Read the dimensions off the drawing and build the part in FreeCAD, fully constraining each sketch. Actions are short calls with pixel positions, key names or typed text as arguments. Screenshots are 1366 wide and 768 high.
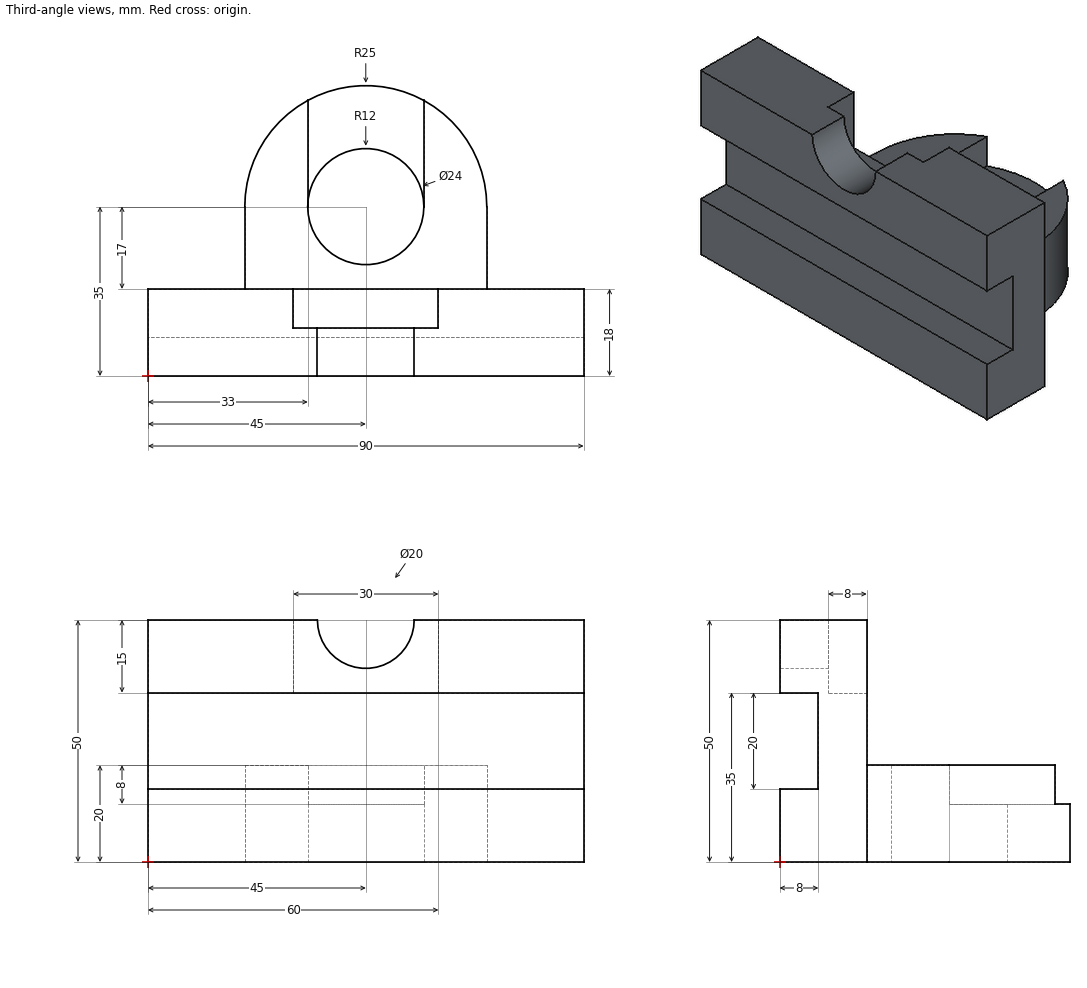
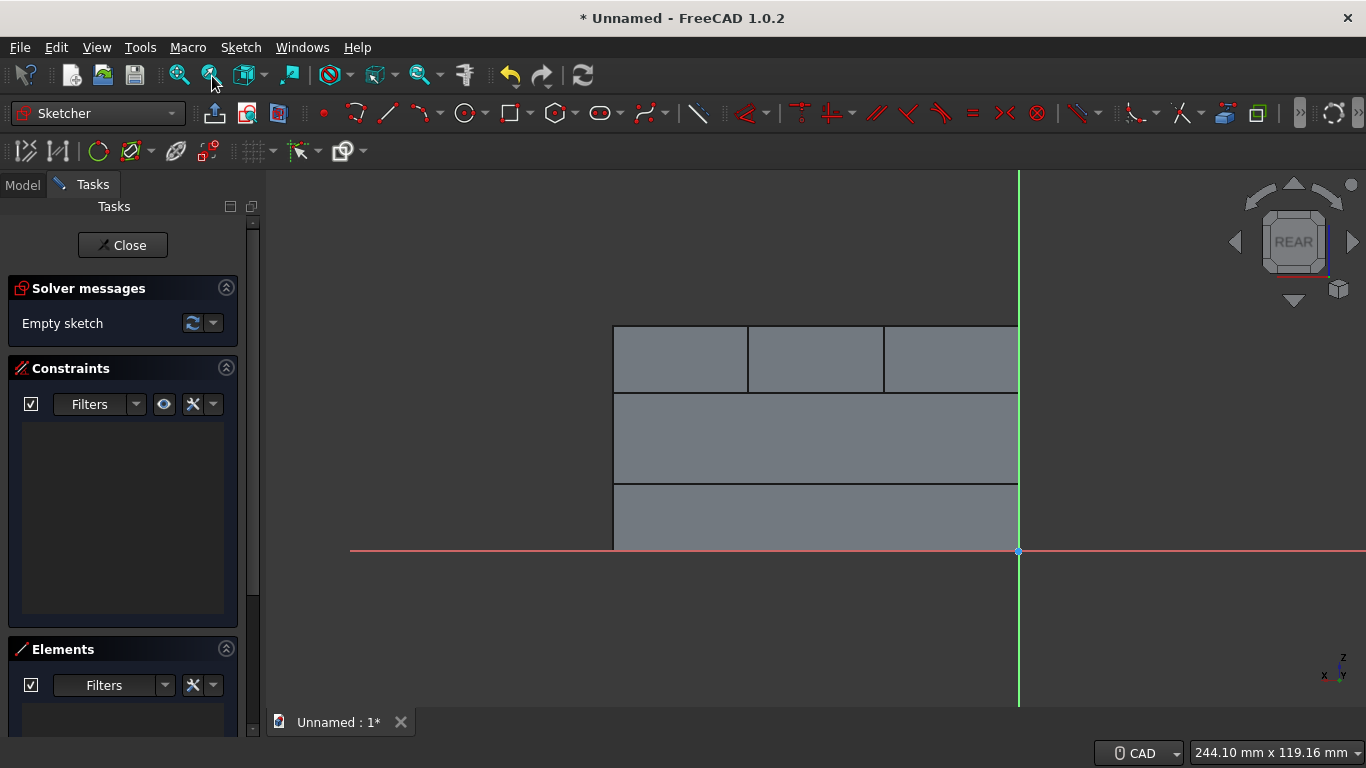
scroll(838, 289, up, 7)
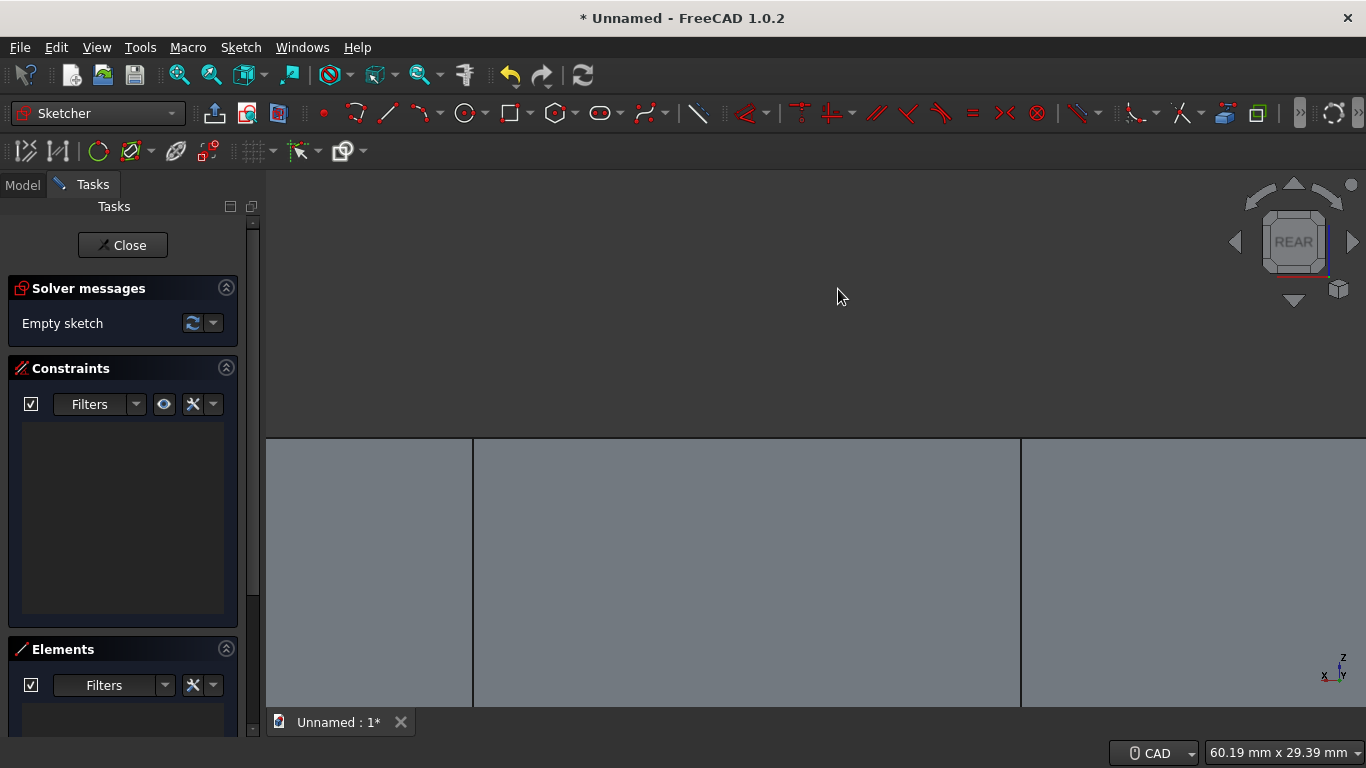
click(466, 114)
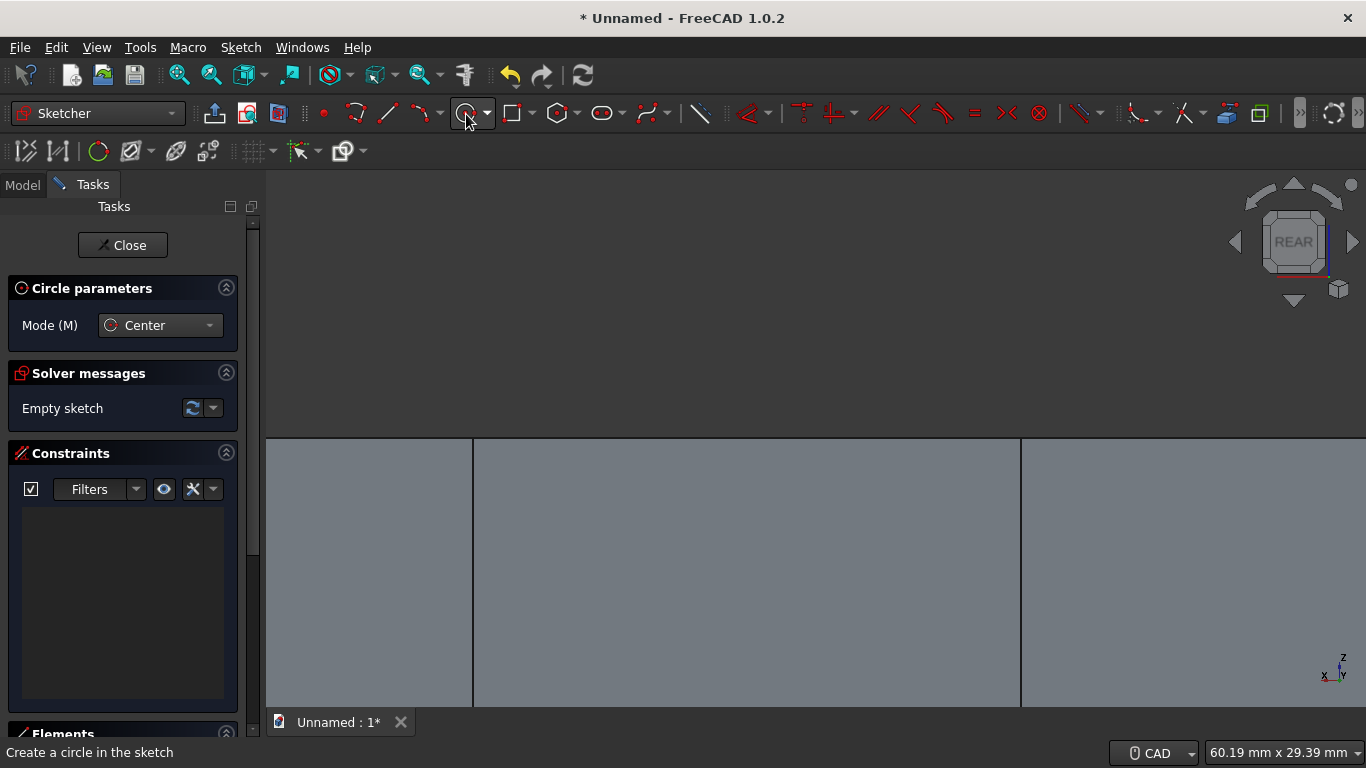
click(747, 438)
move(876, 308)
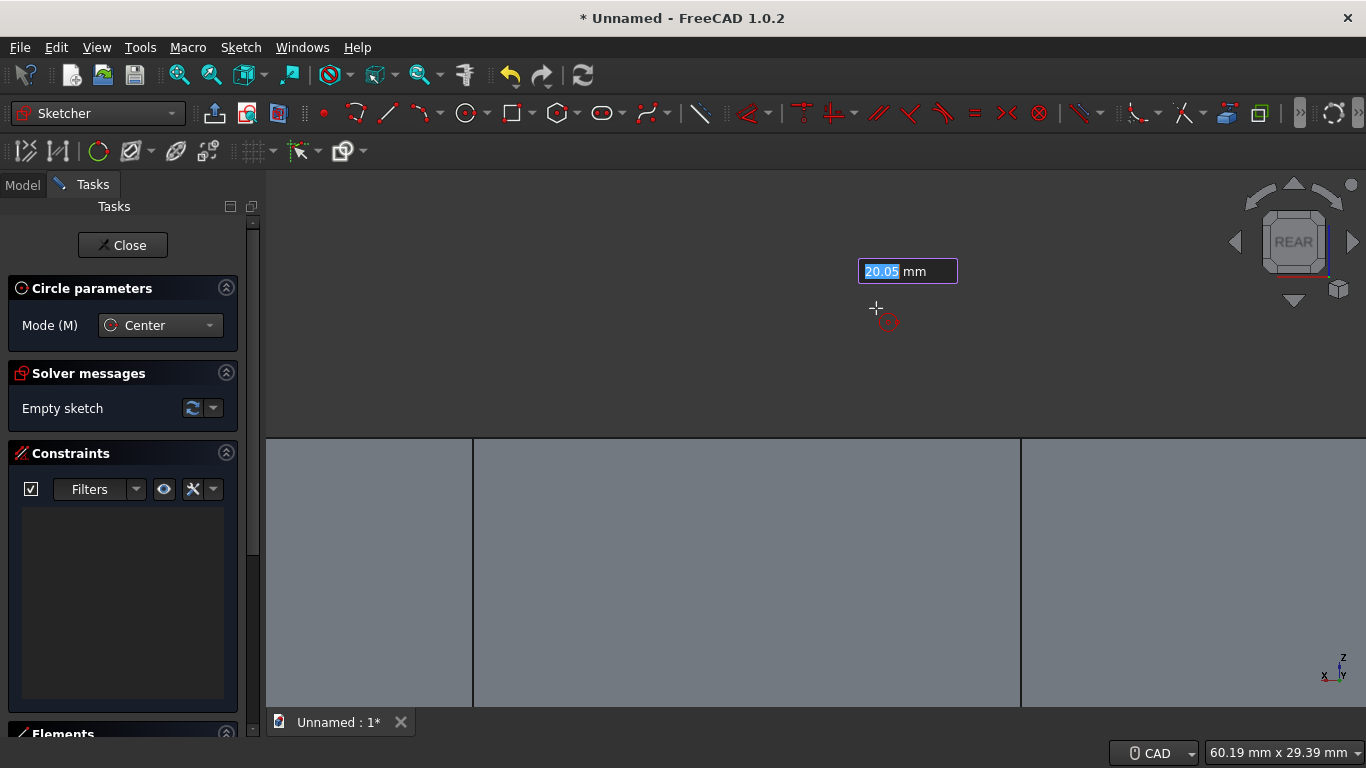
text(20)
key(Return)
key(Escape)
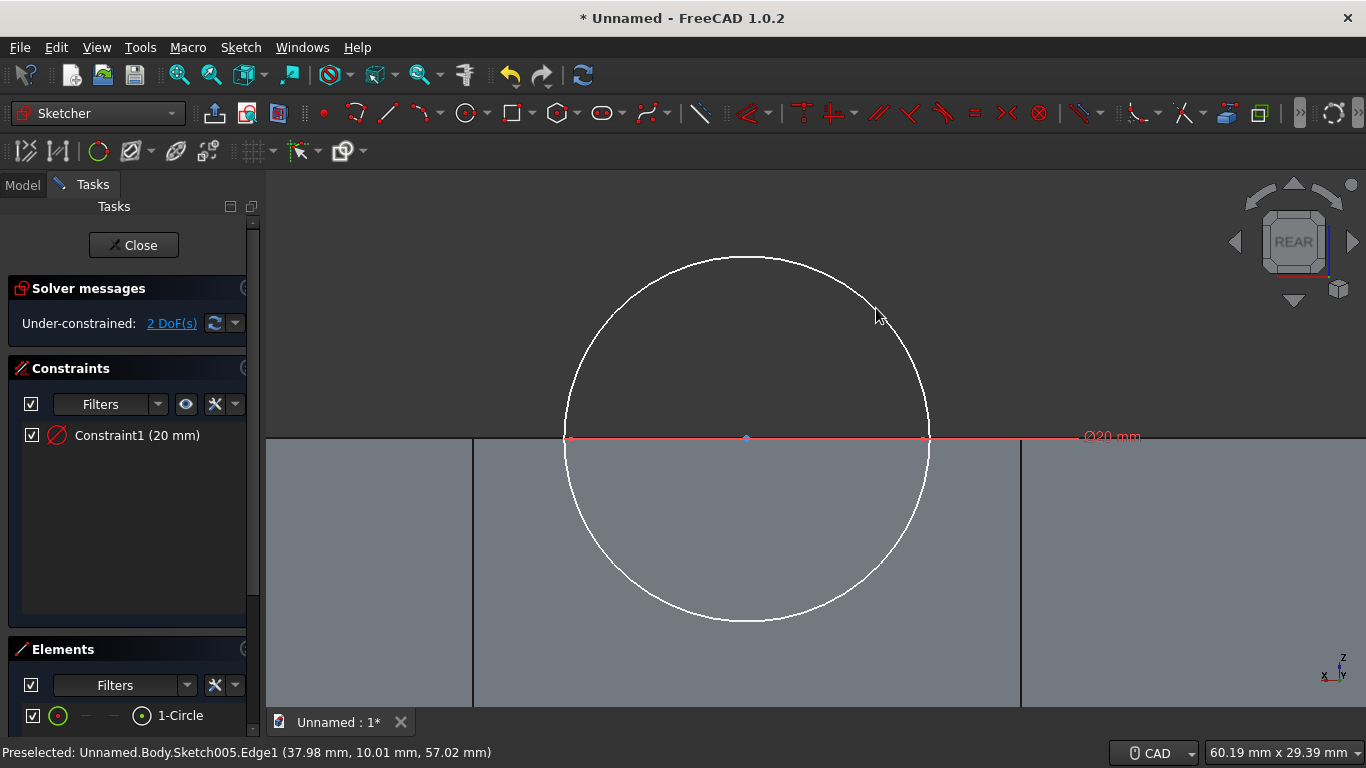
key(d)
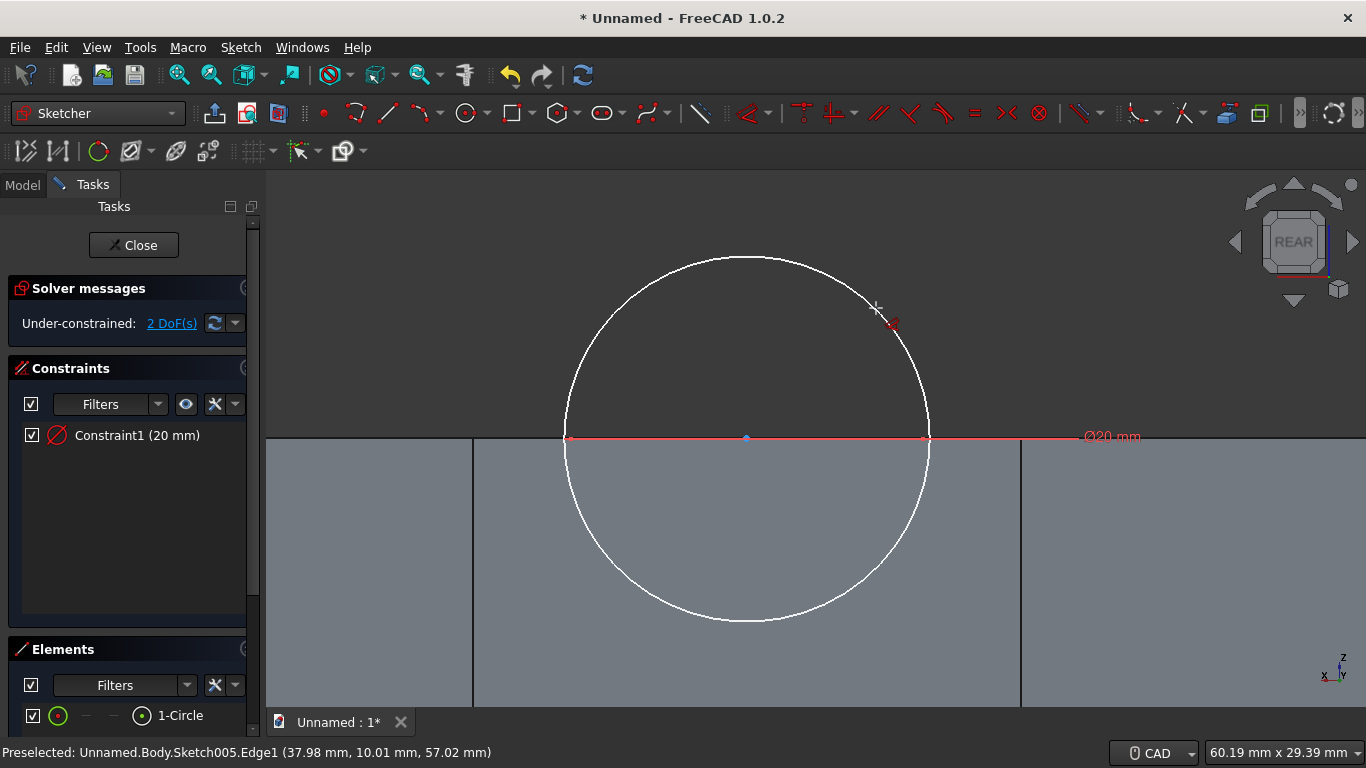
click(747, 439)
click(974, 405)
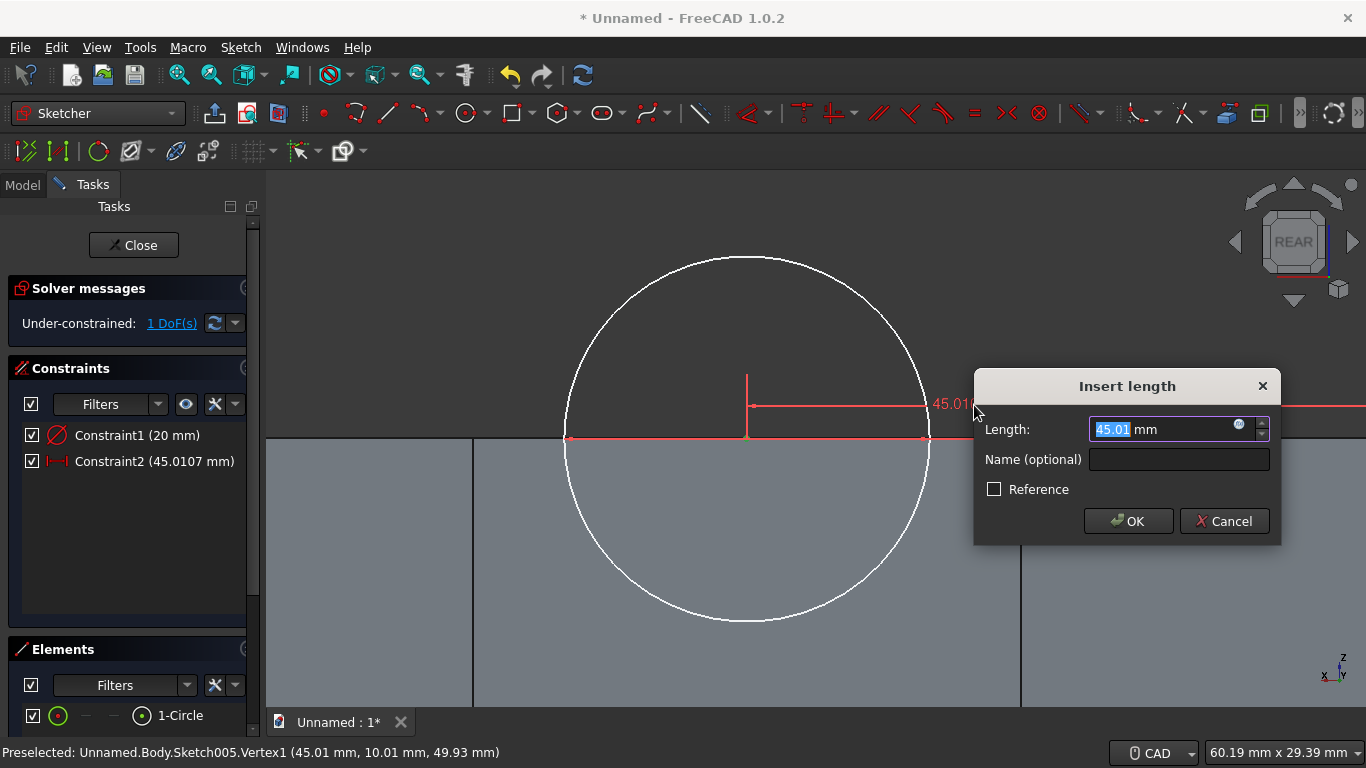
text(45)
key(Return)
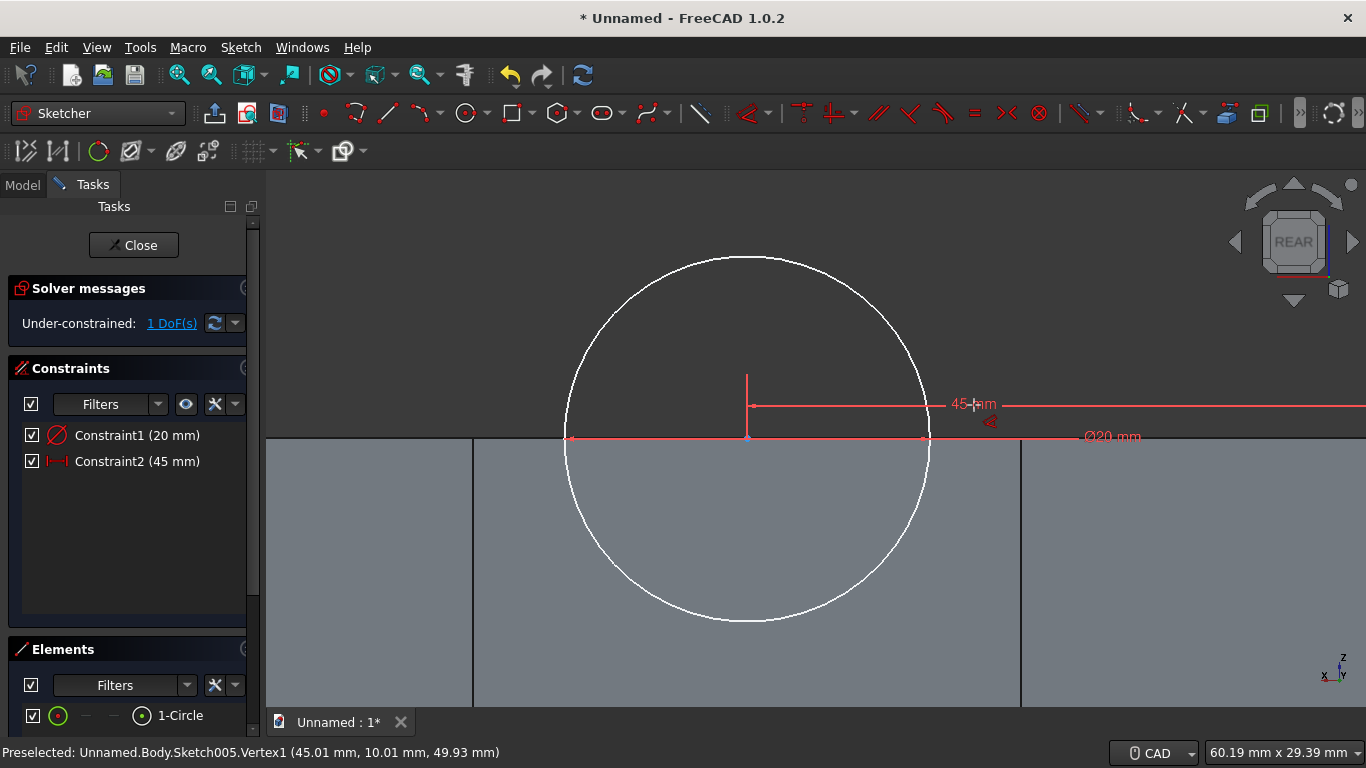
click(747, 439)
click(713, 559)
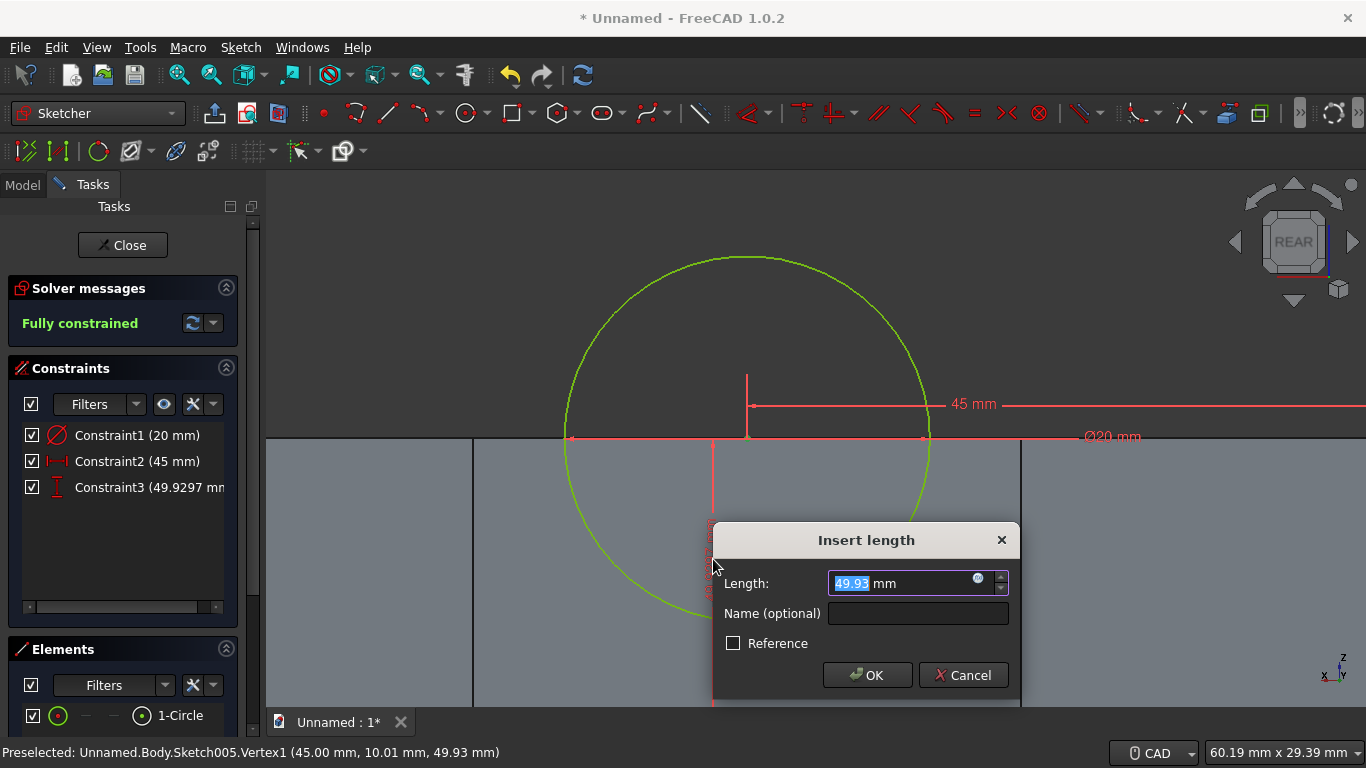
text(50)
key(Return)
key(Escape)